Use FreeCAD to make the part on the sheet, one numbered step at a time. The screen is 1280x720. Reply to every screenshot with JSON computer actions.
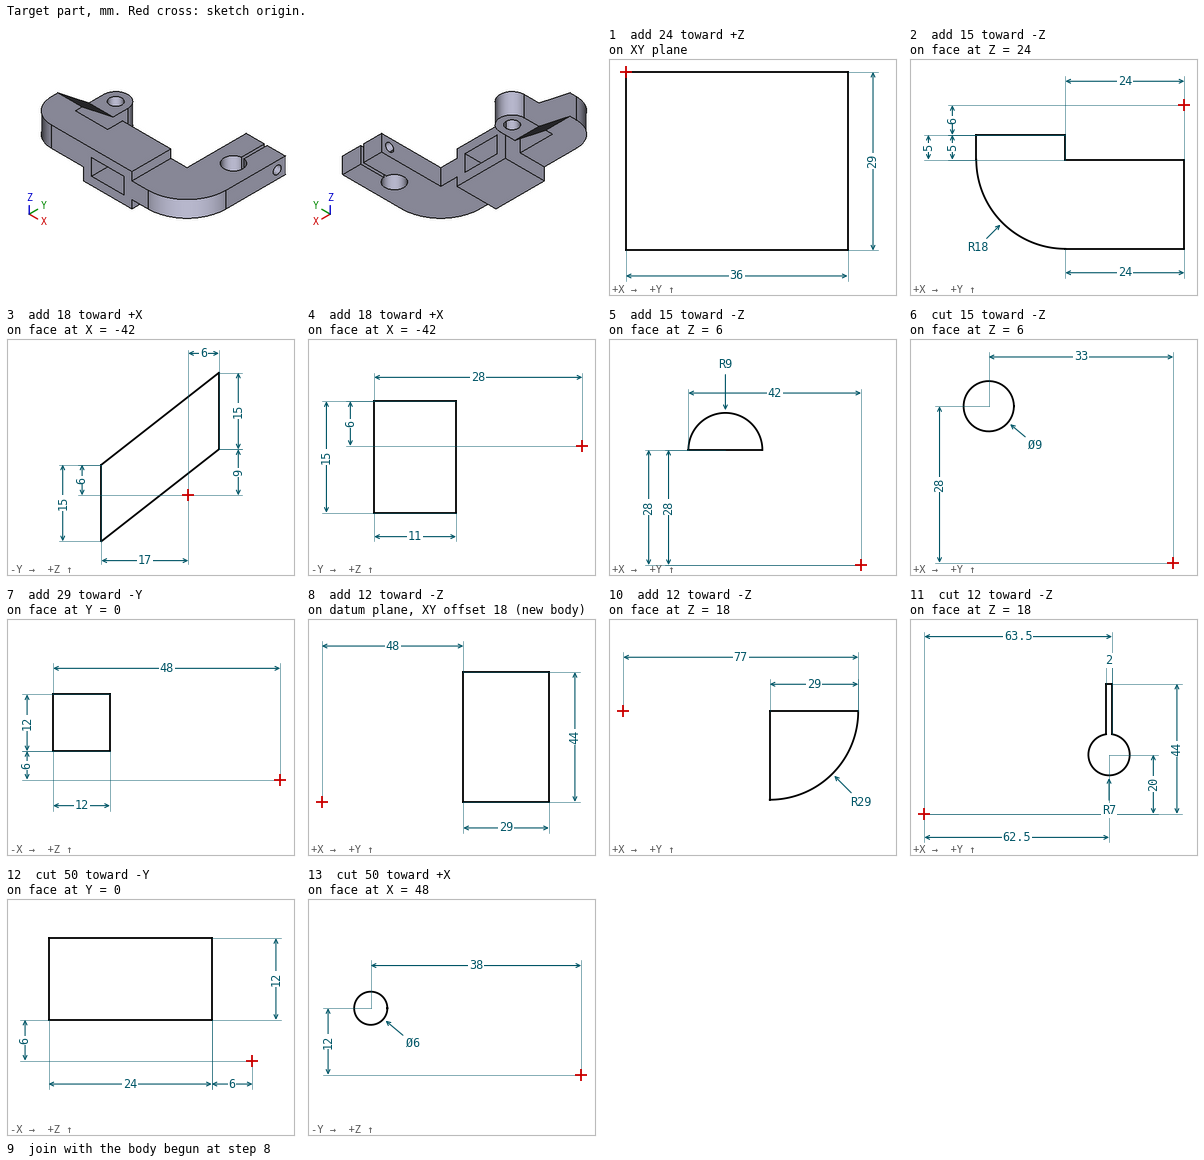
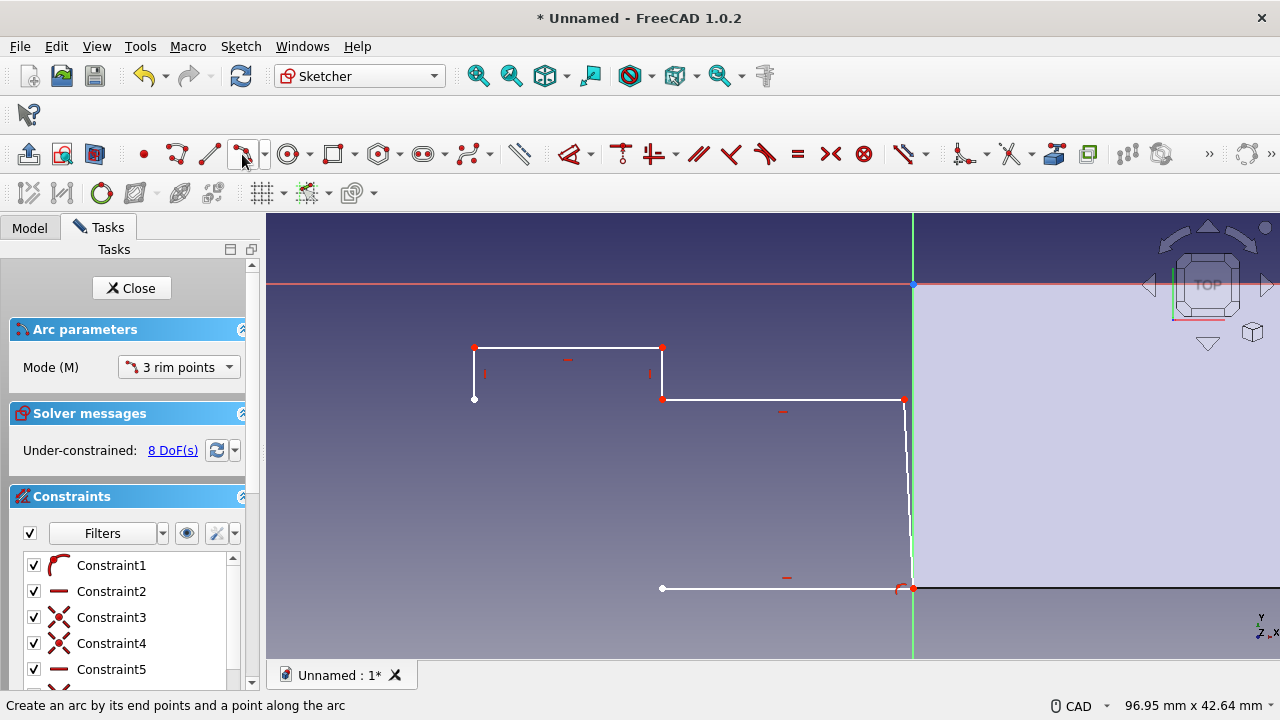
{"action": "left_click", "coordinate": [474, 400]}
{"action": "left_click", "coordinate": [662, 589]}
{"action": "left_click", "coordinate": [529, 532]}
{"action": "key", "text": "Escape"}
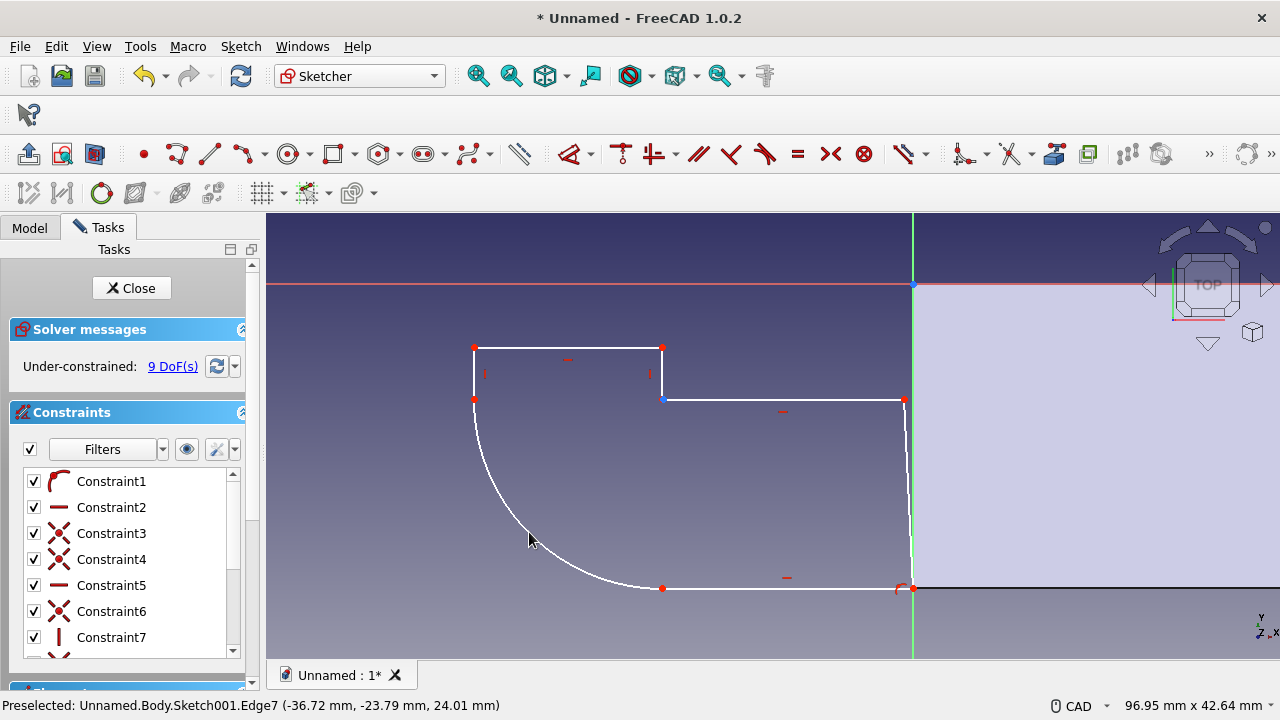
{"action": "left_click", "coordinate": [737, 589]}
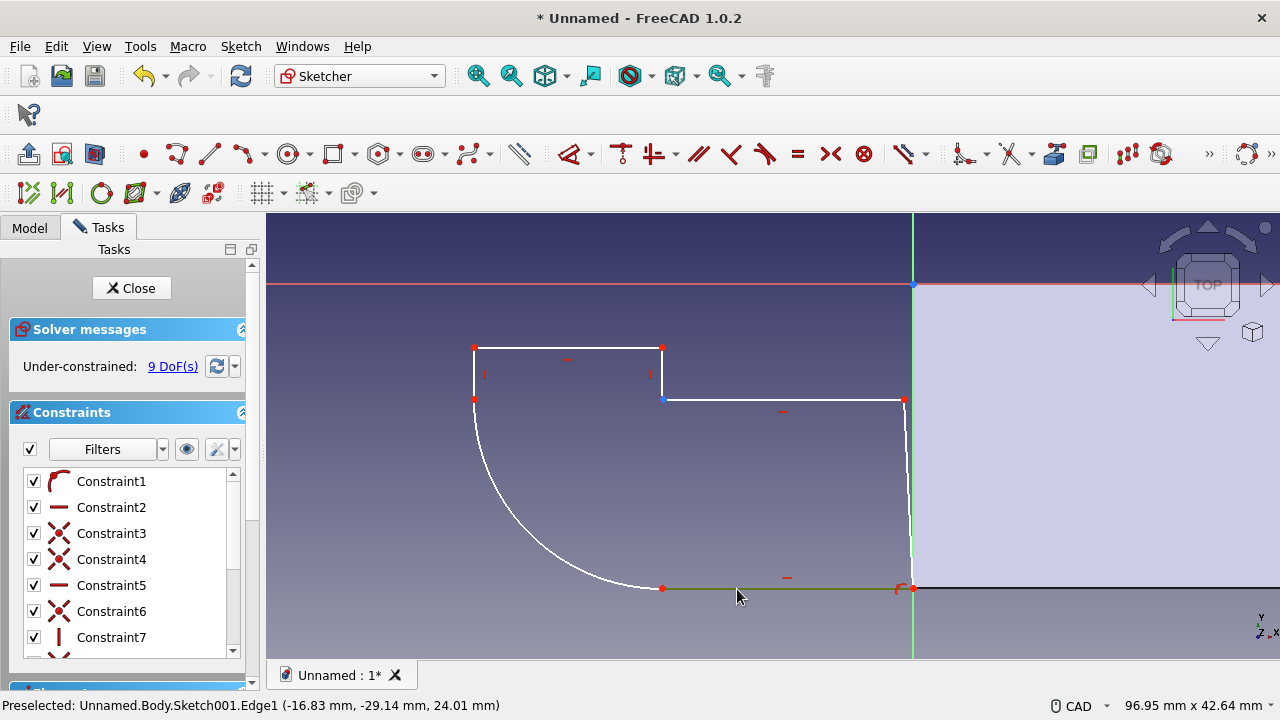
{"action": "left_click", "coordinate": [495, 485]}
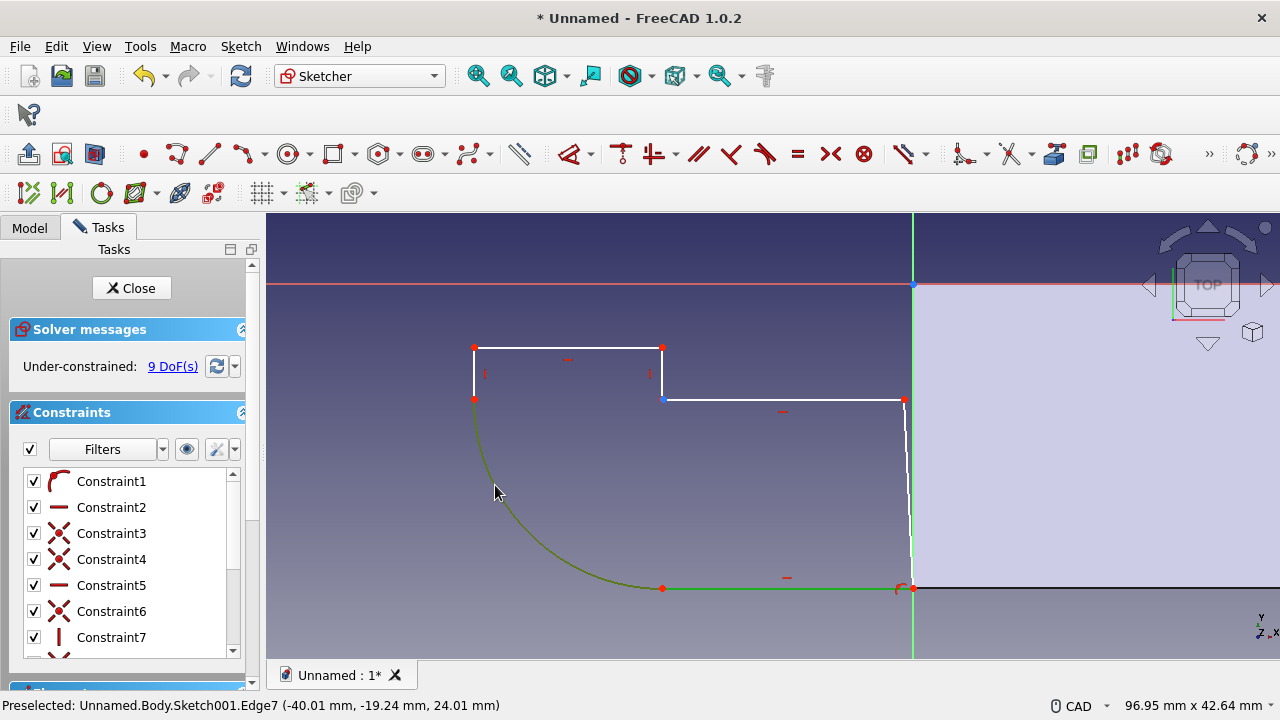
{"action": "left_click", "coordinate": [765, 154]}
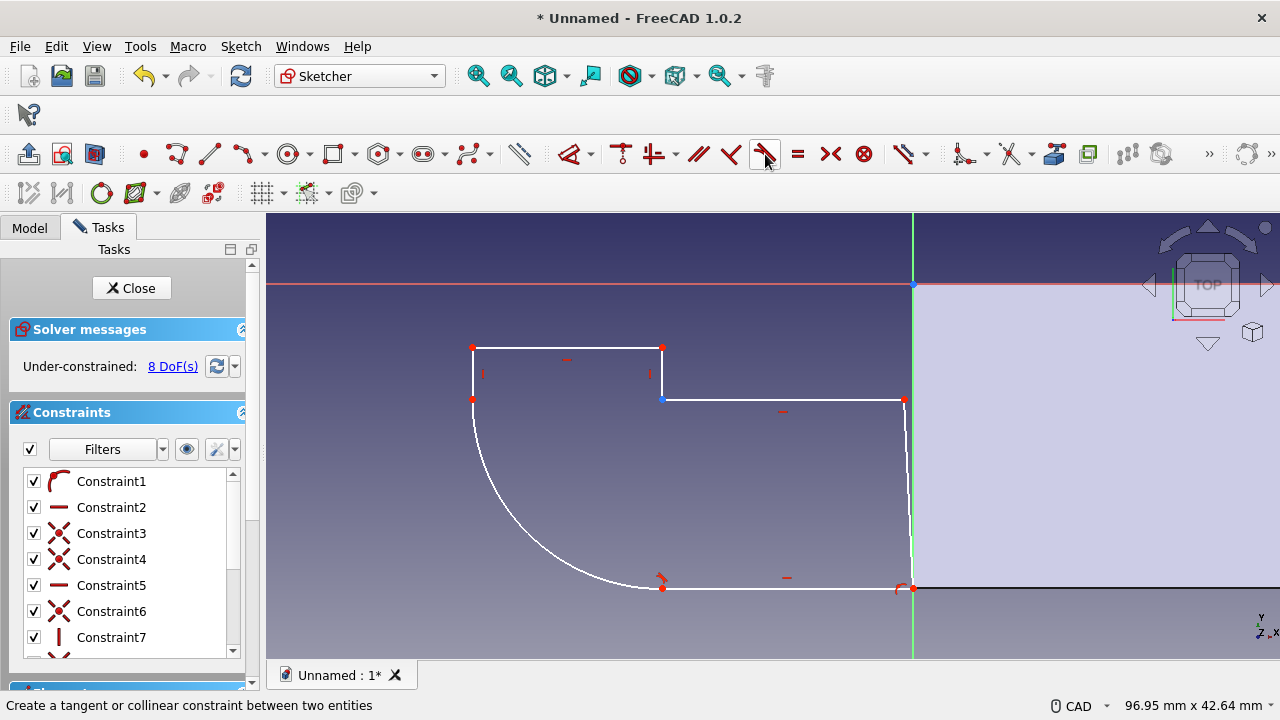
{"action": "left_click", "coordinate": [473, 364]}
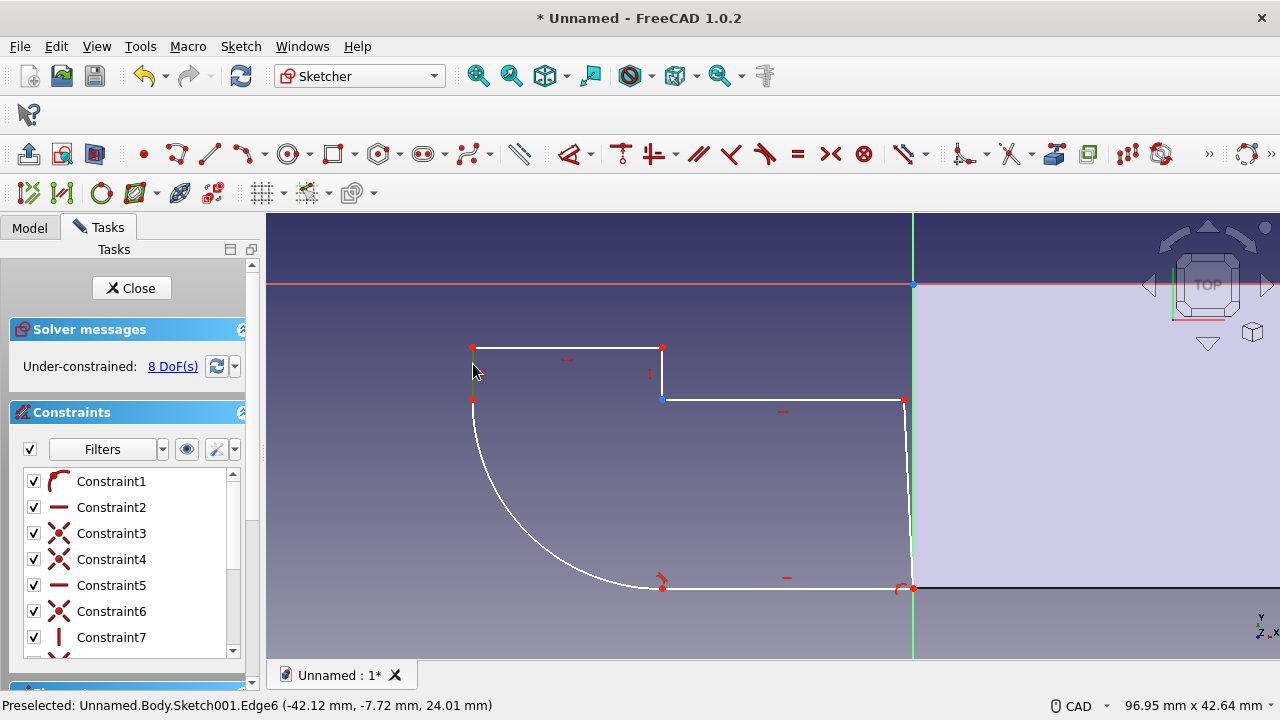
{"action": "left_click", "coordinate": [493, 486]}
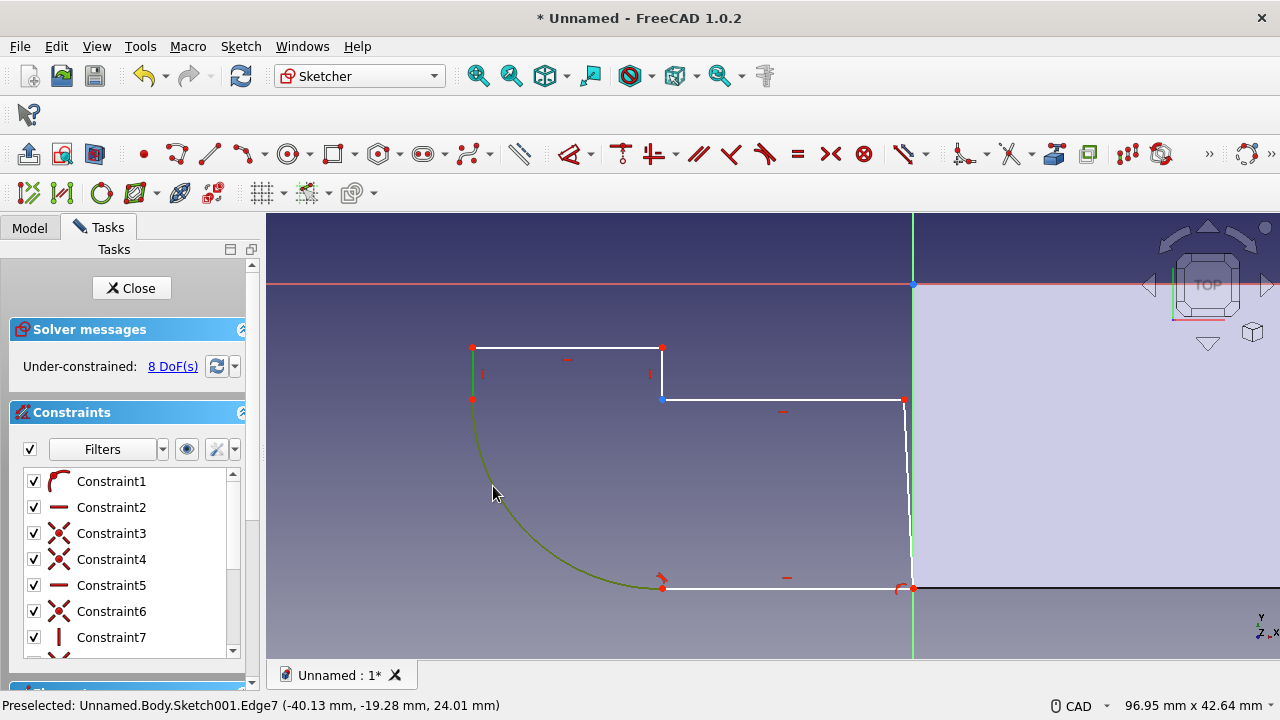
{"action": "left_click", "coordinate": [765, 154]}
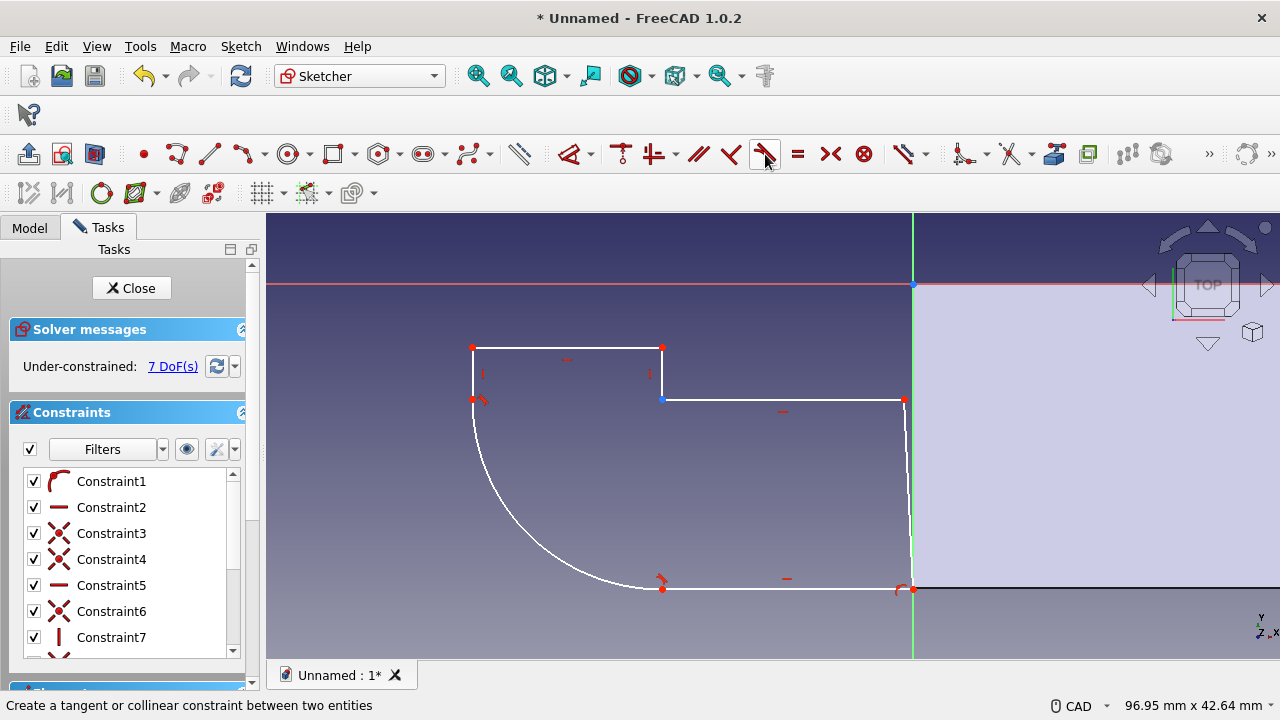
{"action": "left_click", "coordinate": [910, 533]}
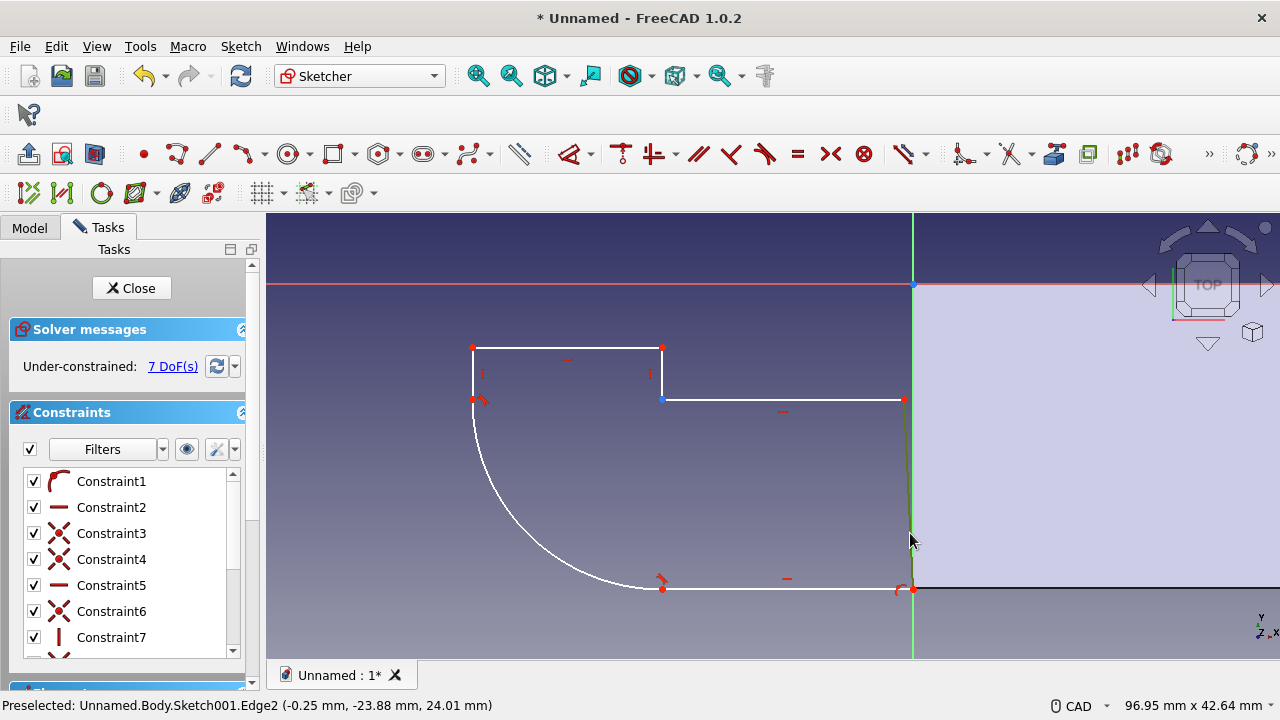
{"action": "left_click", "coordinate": [676, 154]}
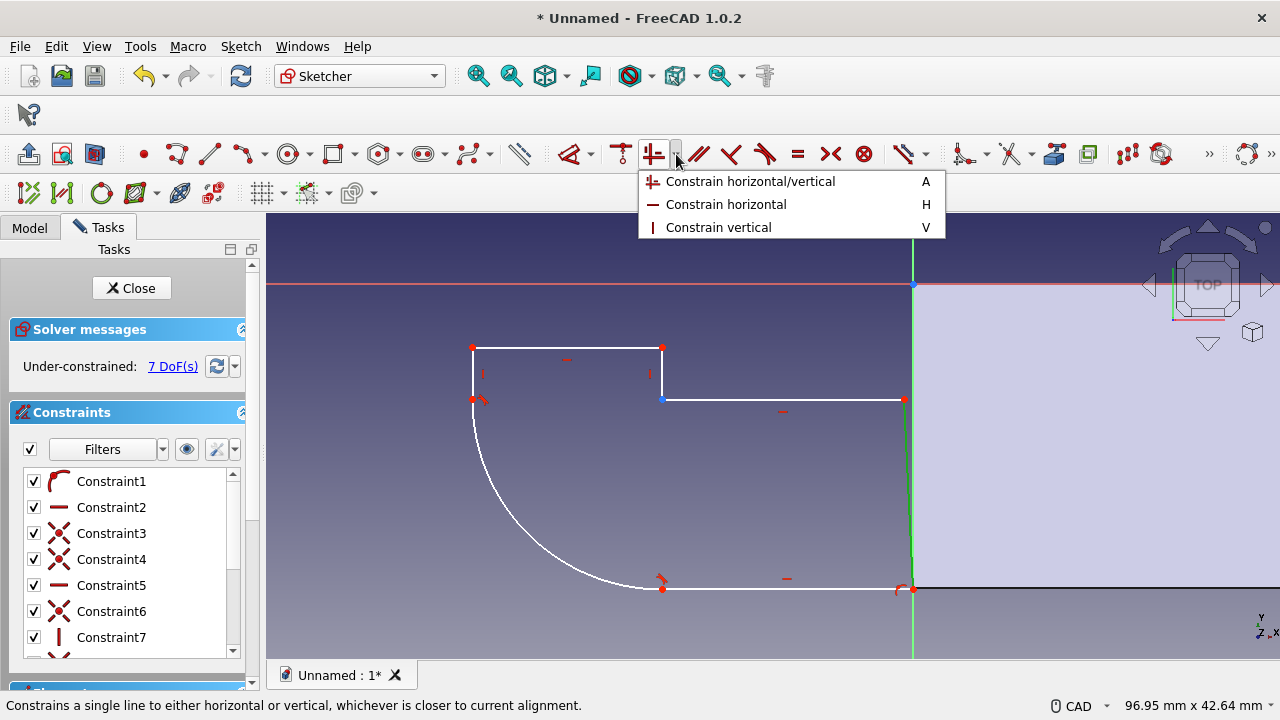
{"action": "left_click", "coordinate": [792, 228]}